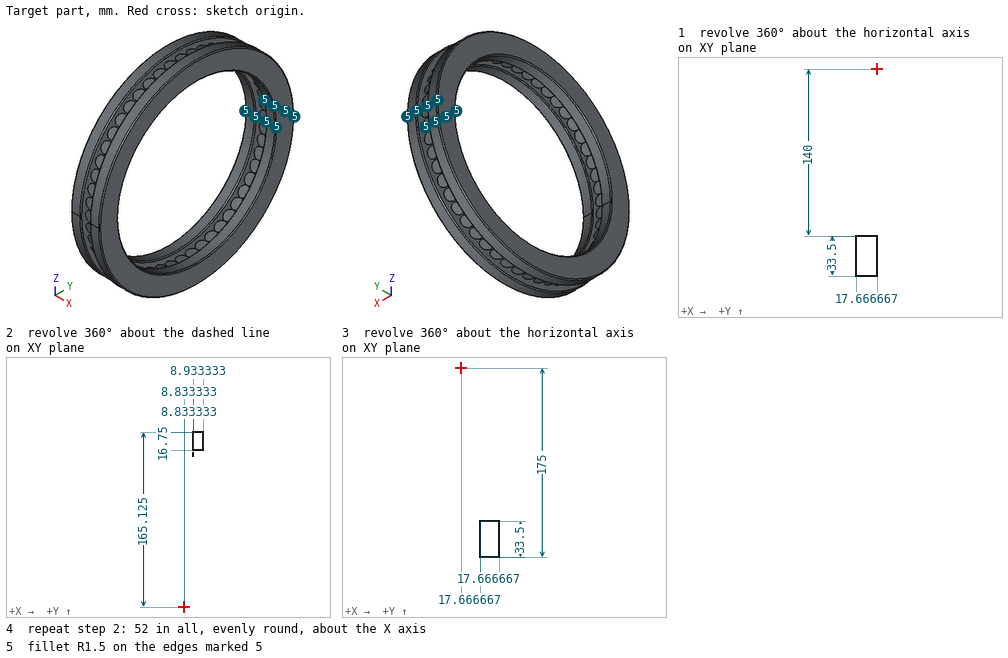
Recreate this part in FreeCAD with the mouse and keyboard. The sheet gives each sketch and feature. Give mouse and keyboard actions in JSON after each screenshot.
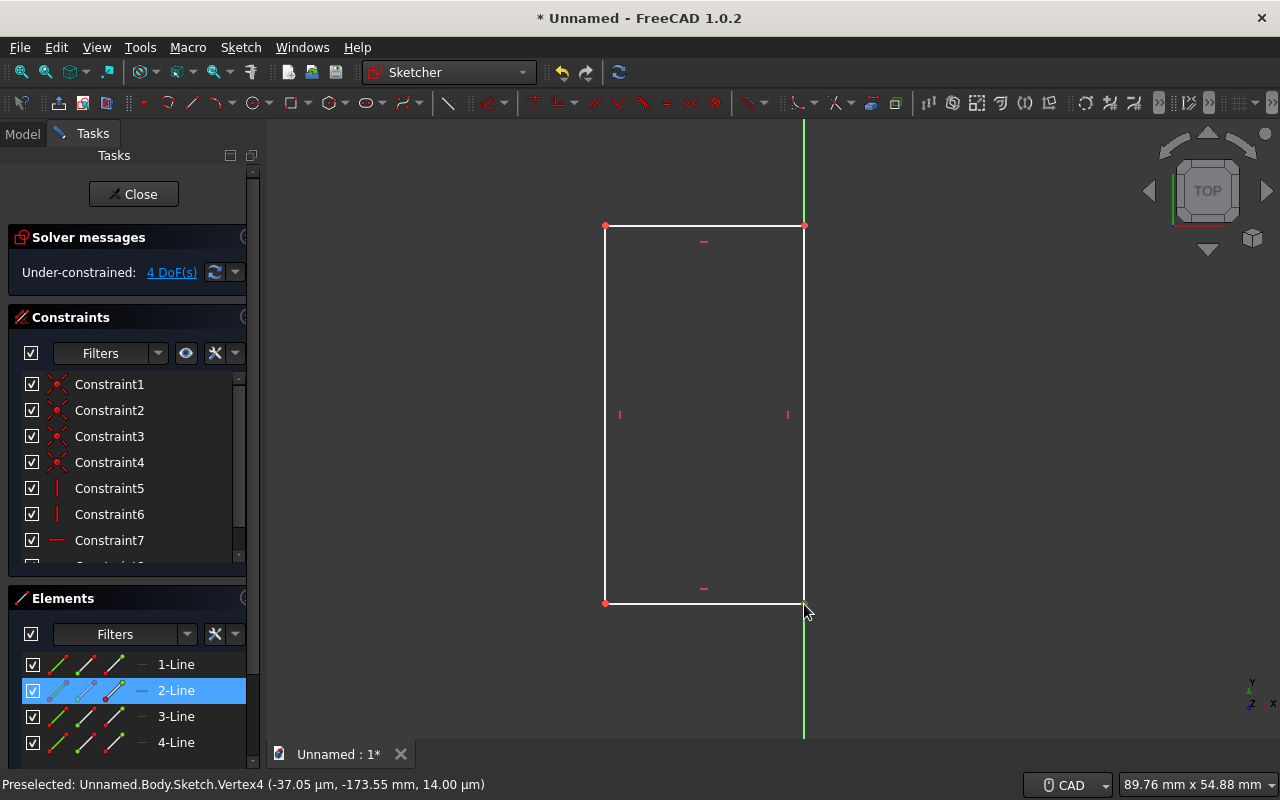
{"action": "left_click", "coordinate": [804, 671]}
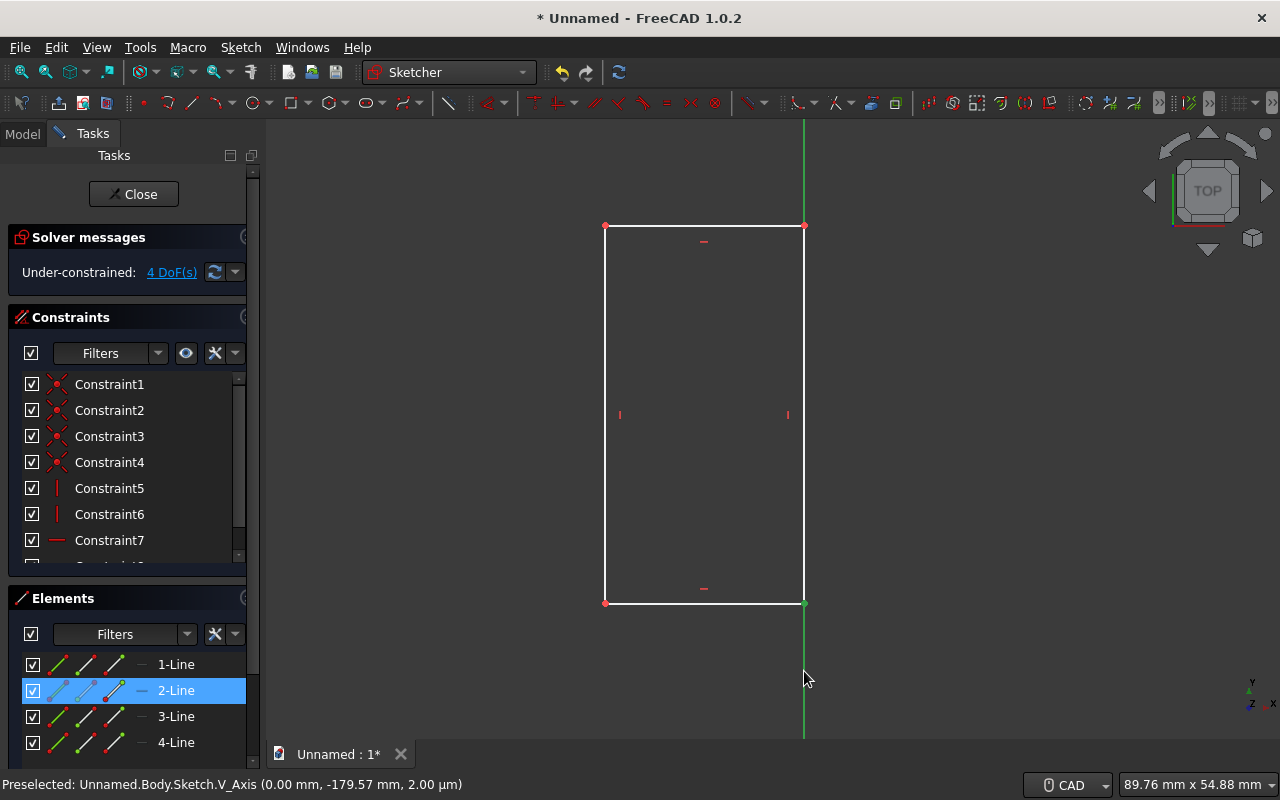
{"action": "left_click", "coordinate": [534, 104]}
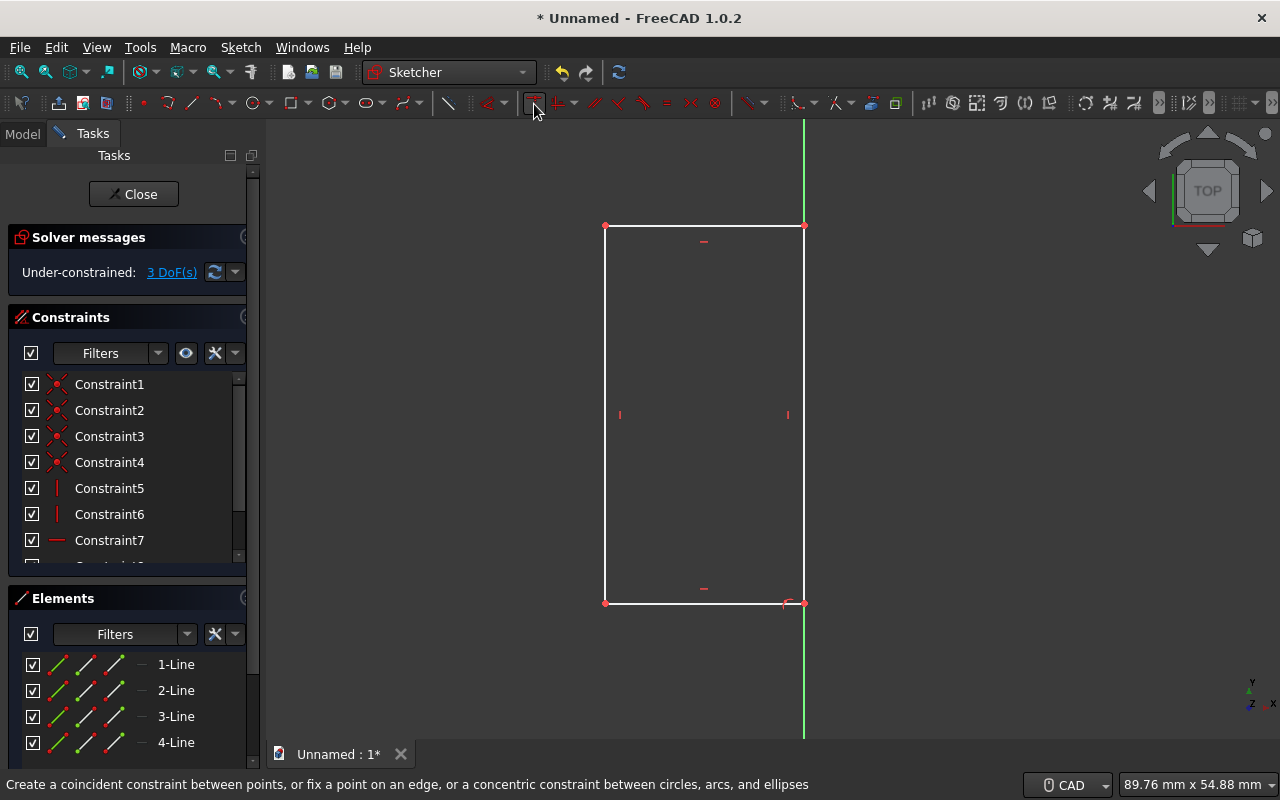
{"action": "left_click", "coordinate": [488, 104]}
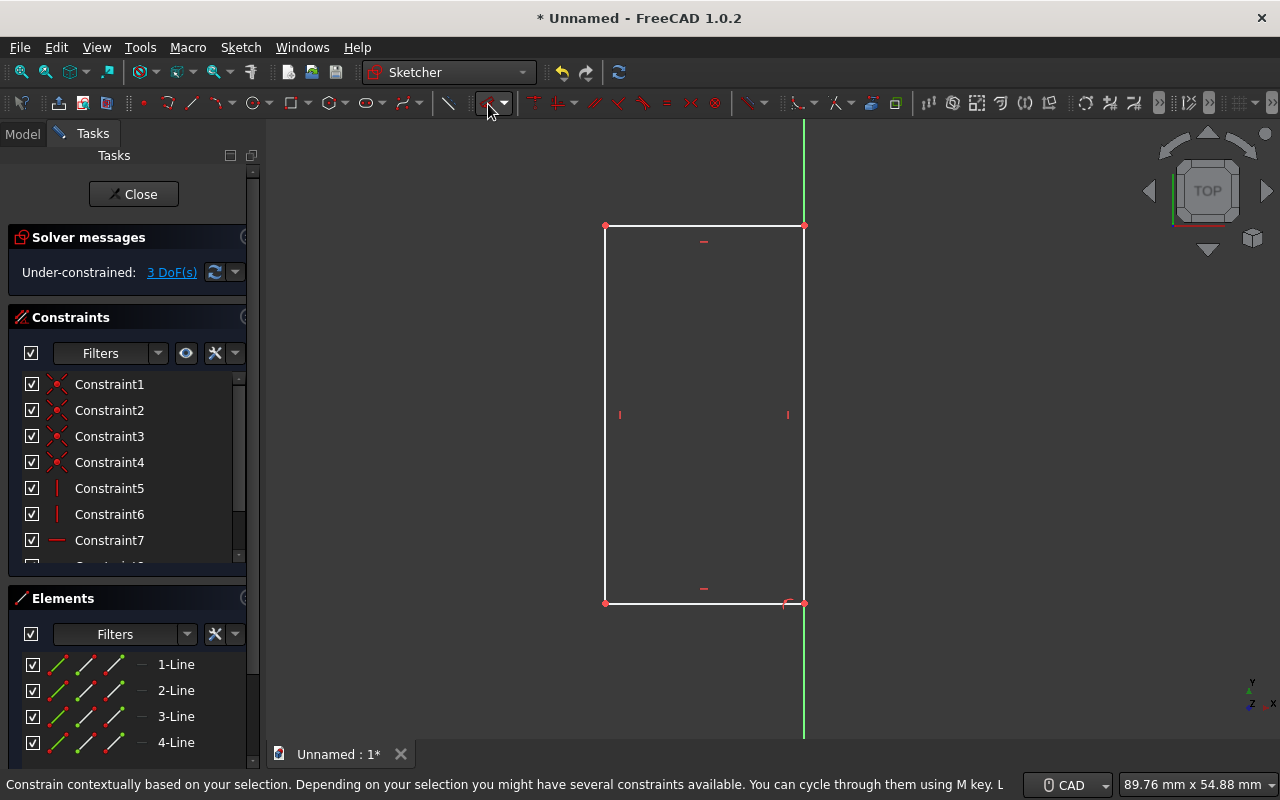
{"action": "left_click", "coordinate": [605, 339]}
{"action": "left_click", "coordinate": [571, 415]}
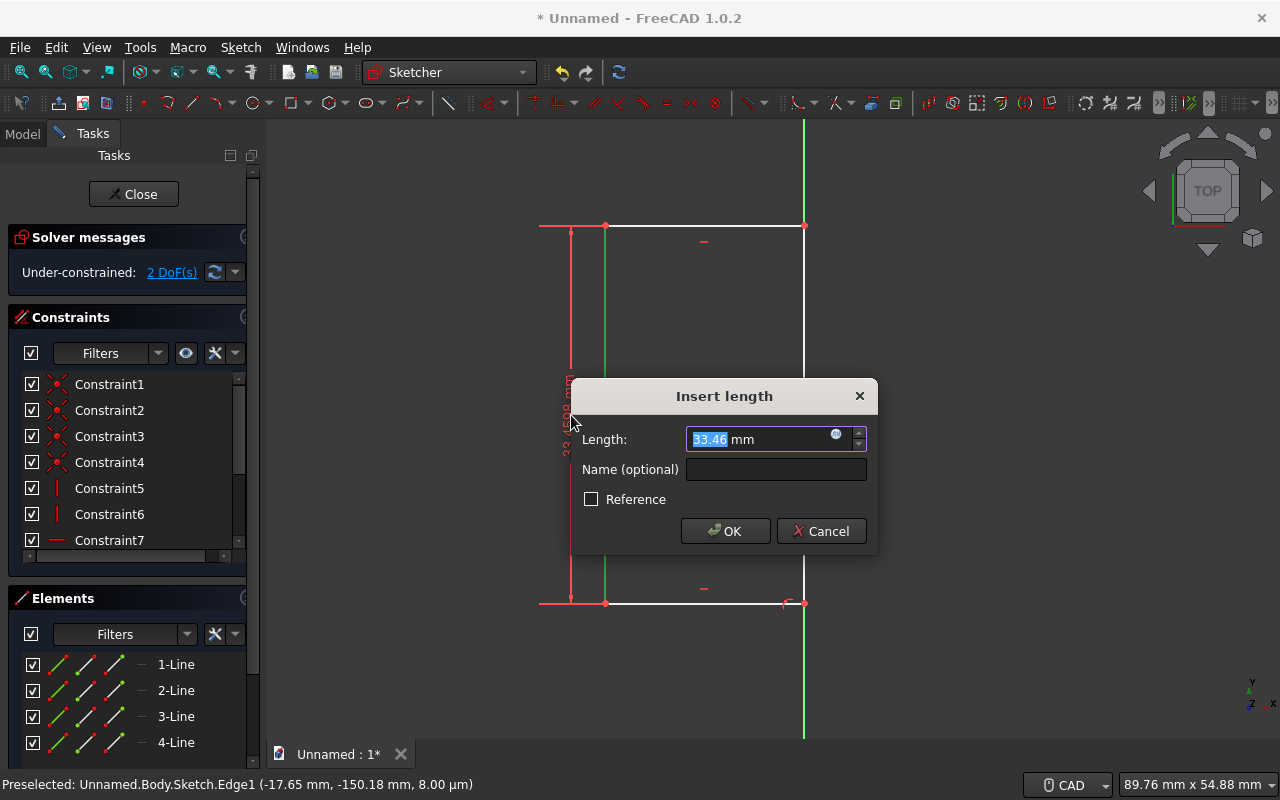
{"action": "type", "text": "33.5"}
{"action": "key", "text": "Return"}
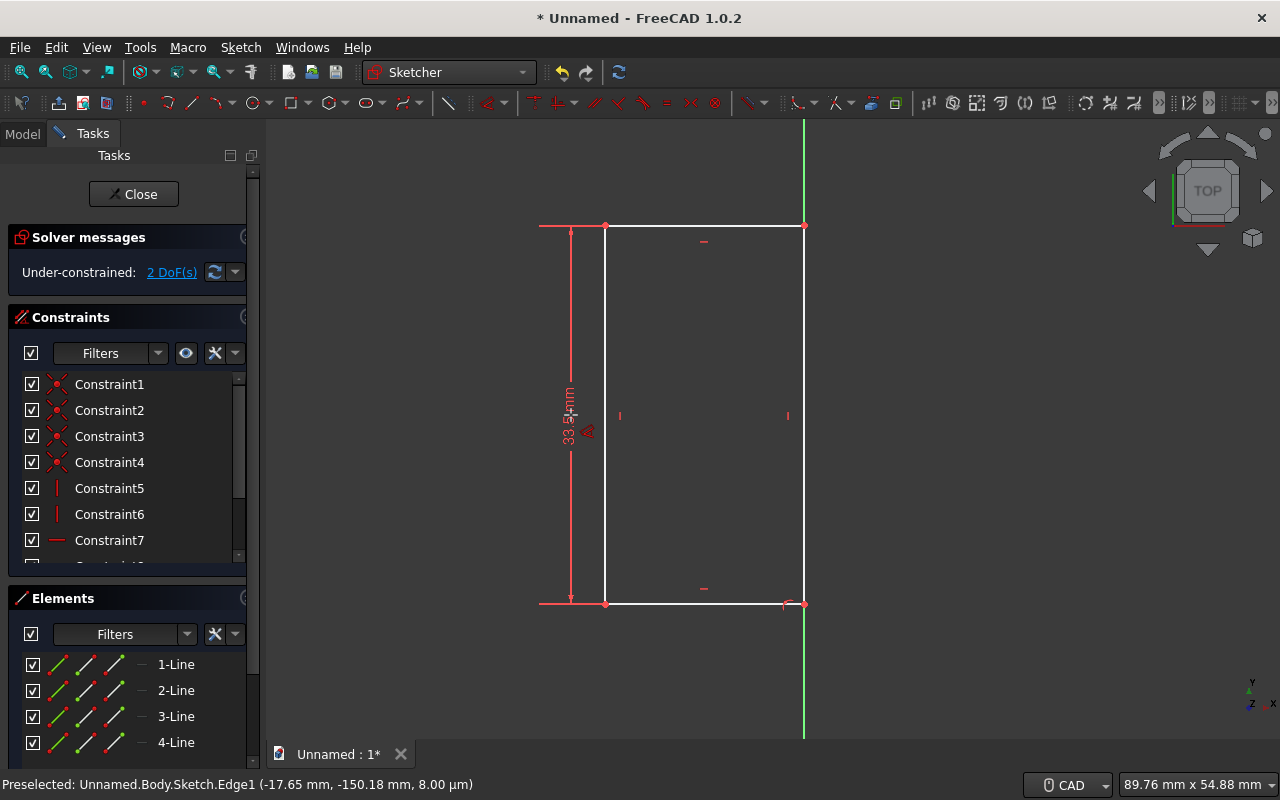
{"action": "left_click", "coordinate": [605, 226]}
{"action": "left_click", "coordinate": [838, 186]}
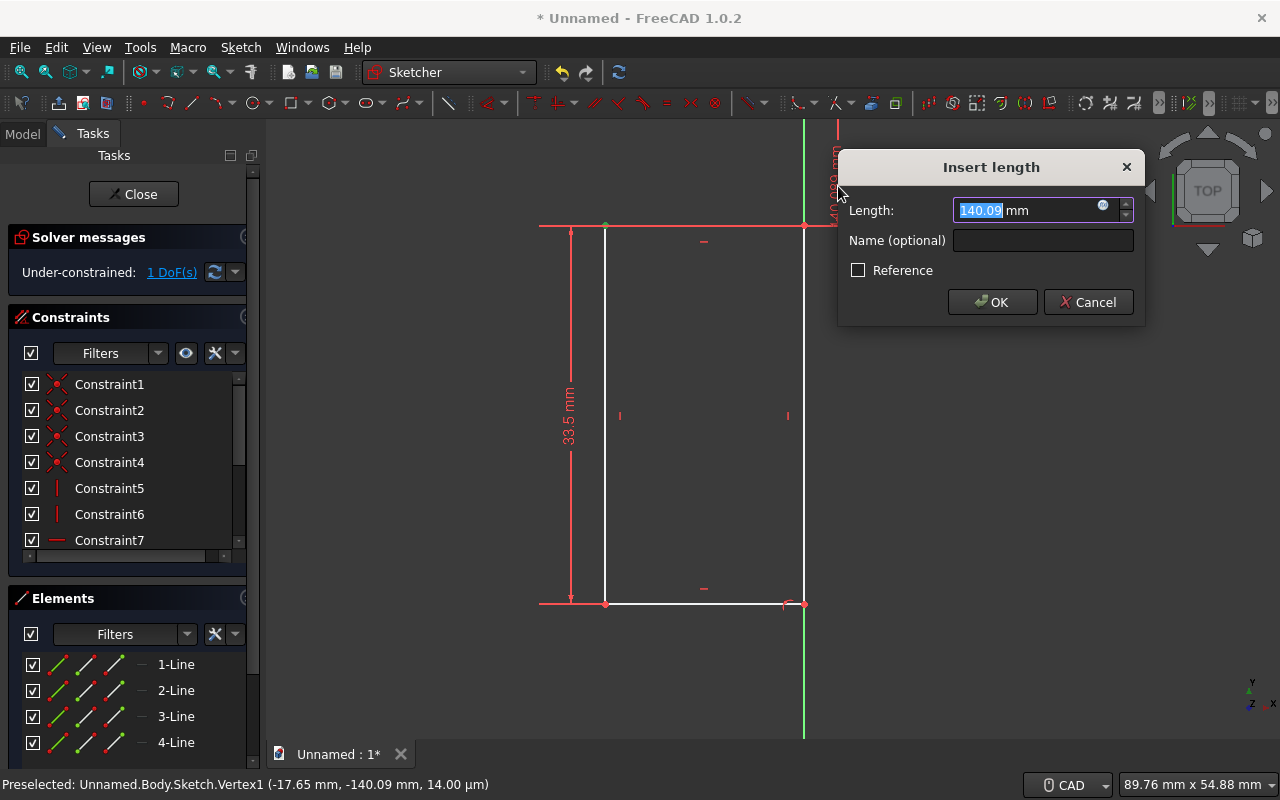
{"action": "type", "text": "140"}
{"action": "key", "text": "Return"}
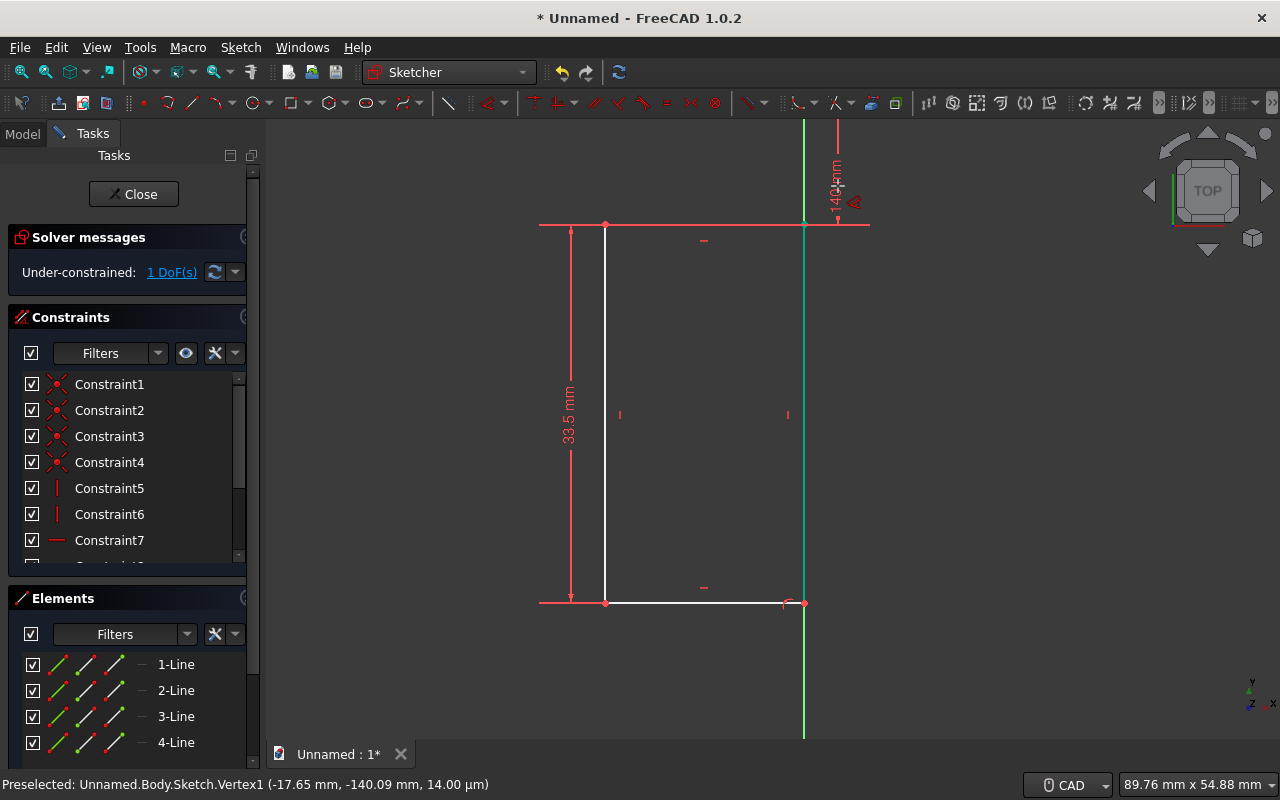
{"action": "left_click", "coordinate": [665, 603]}
{"action": "left_click", "coordinate": [705, 637]}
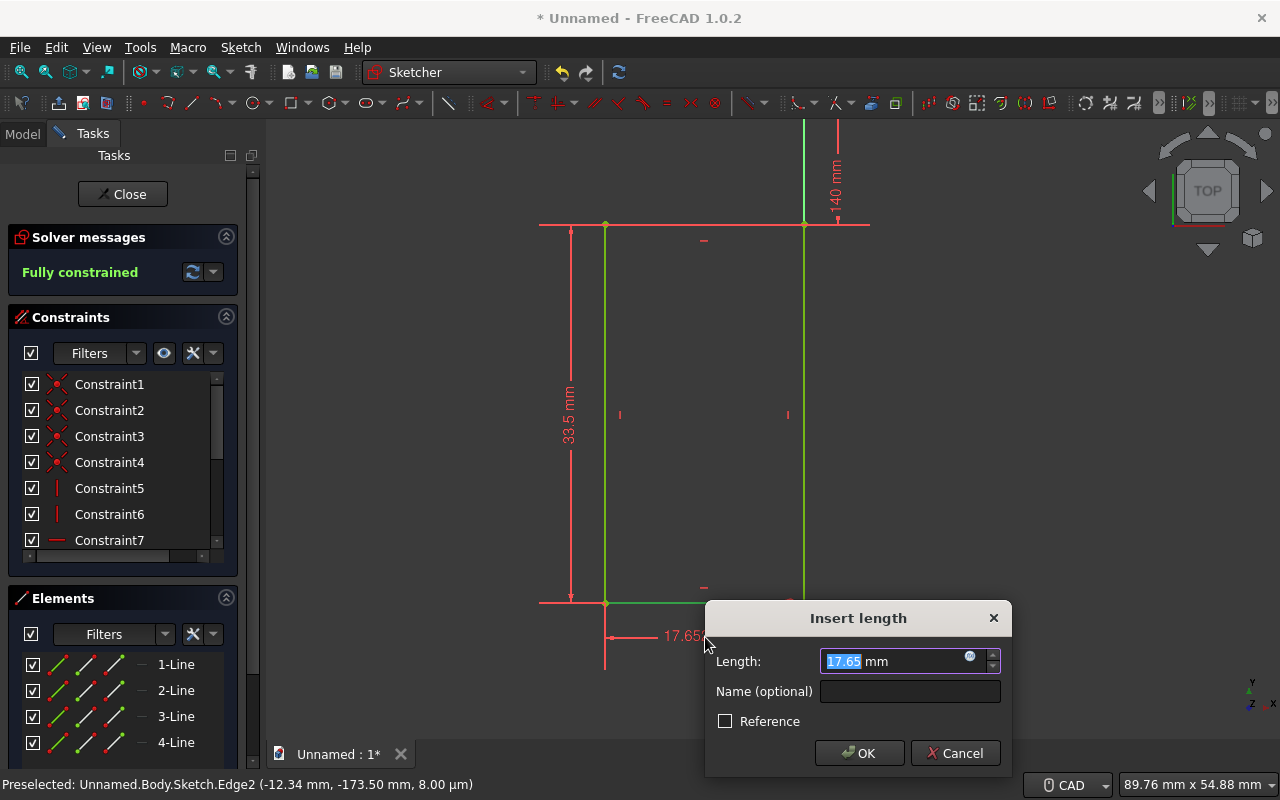
{"action": "type", "text": "17.666667"}
{"action": "key", "text": "Return"}
{"action": "key", "text": "Escape"}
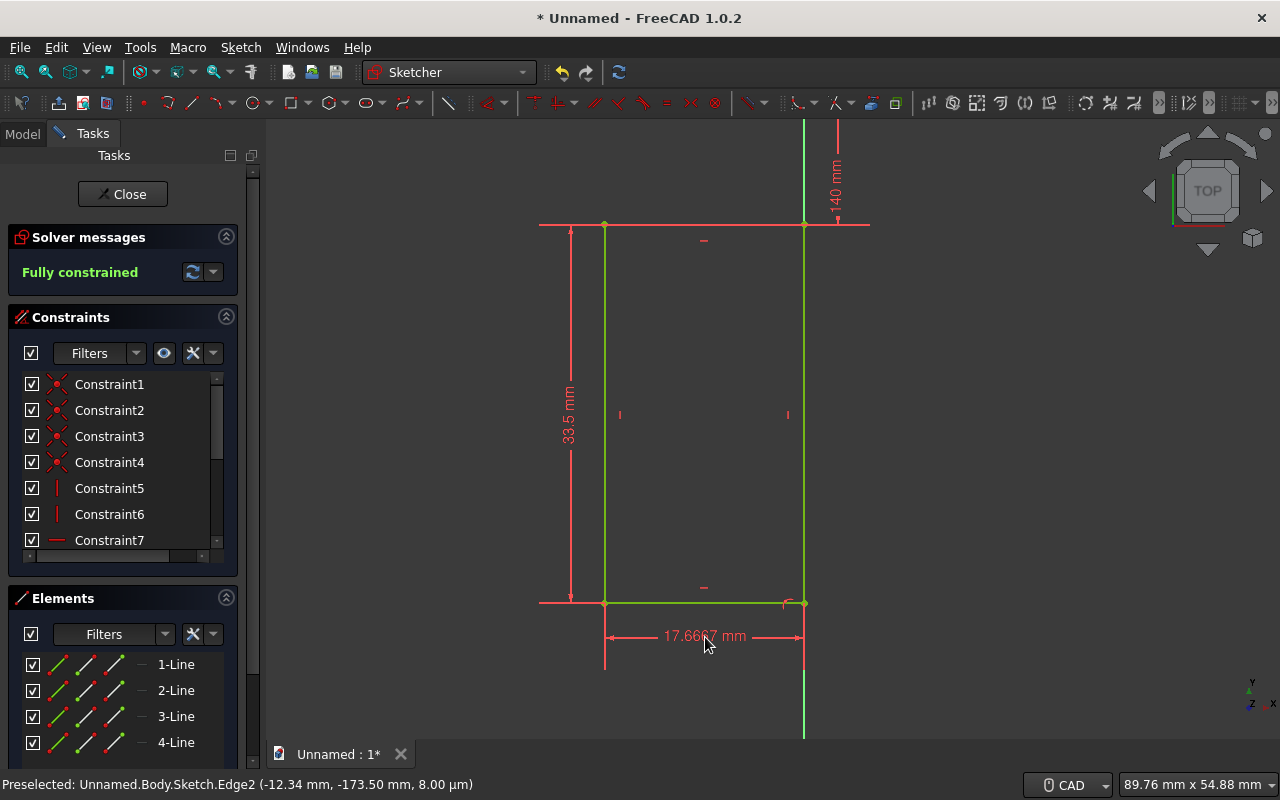
{"action": "left_click", "coordinate": [123, 194]}